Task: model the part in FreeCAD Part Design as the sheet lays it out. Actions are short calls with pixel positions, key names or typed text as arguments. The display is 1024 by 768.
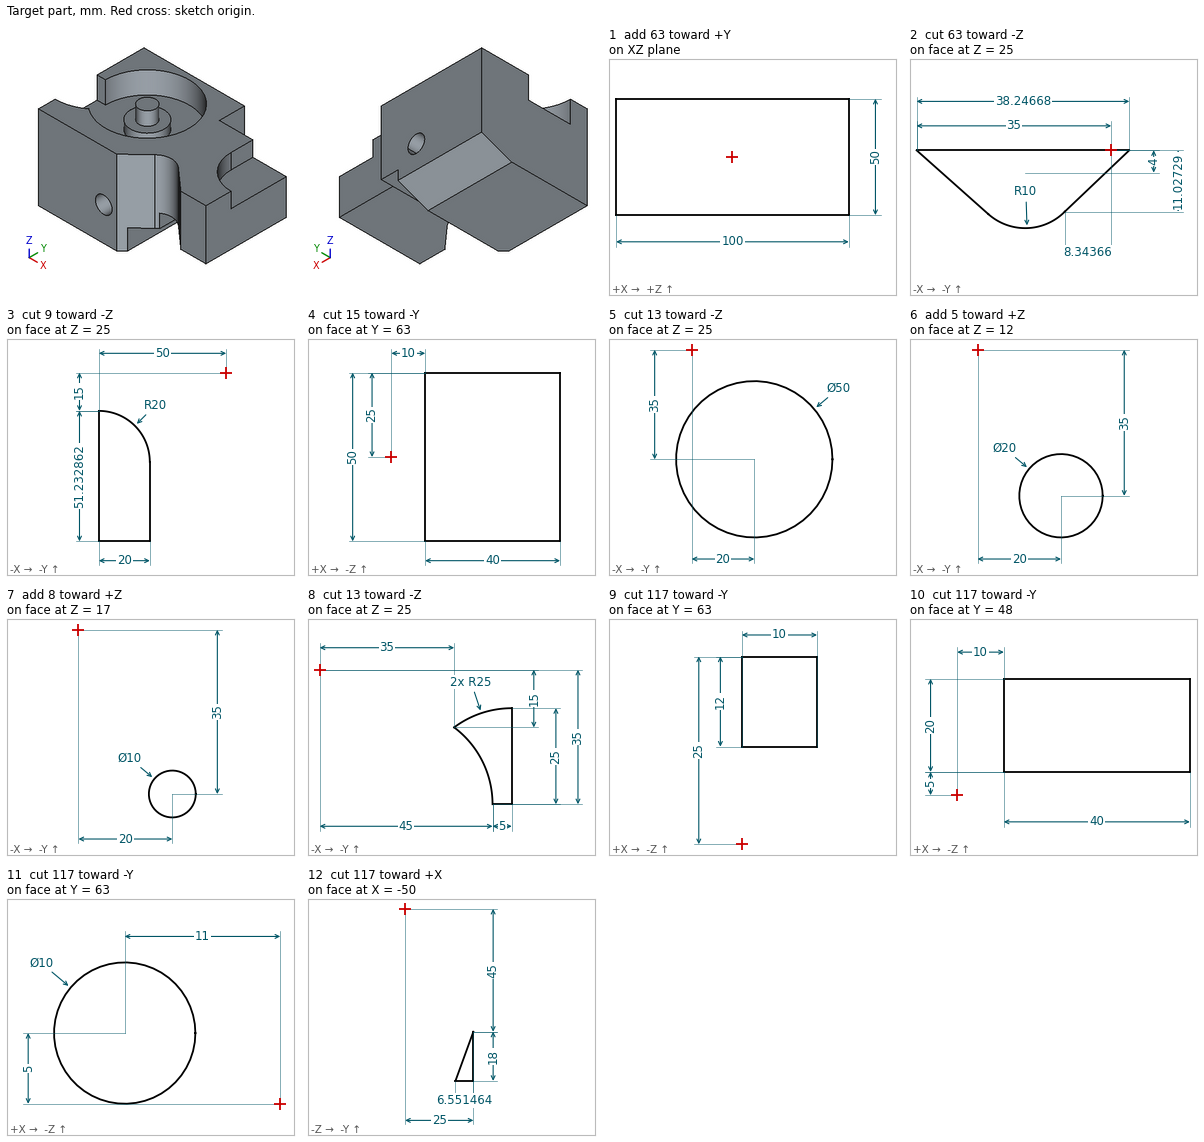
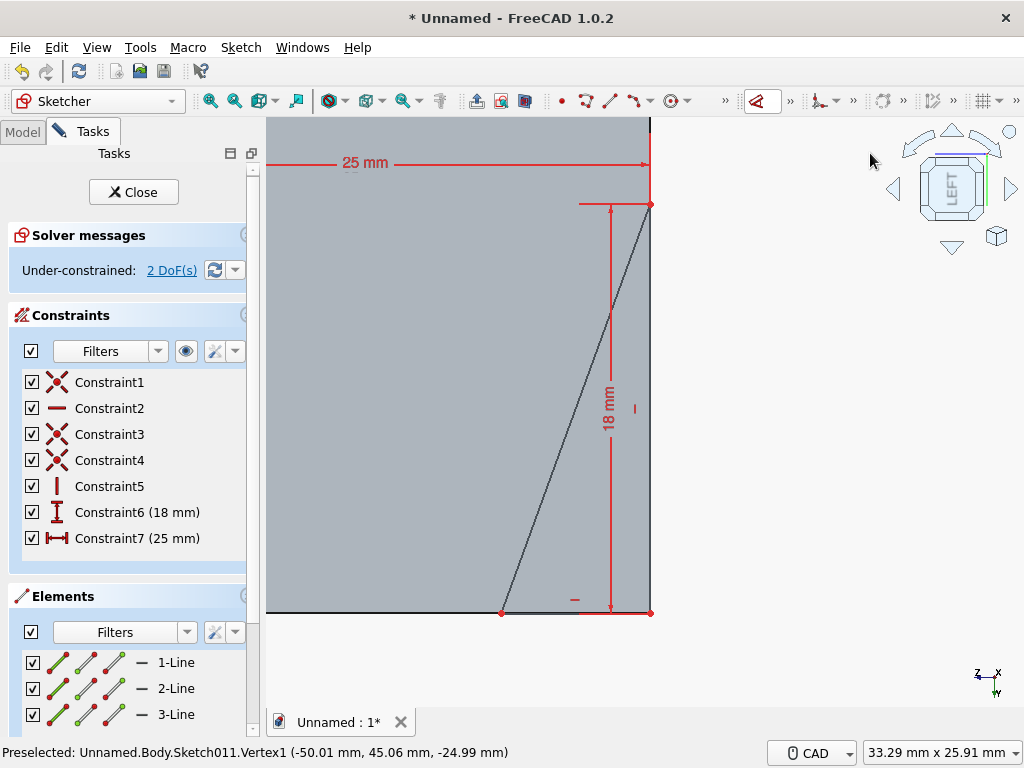
click(650, 204)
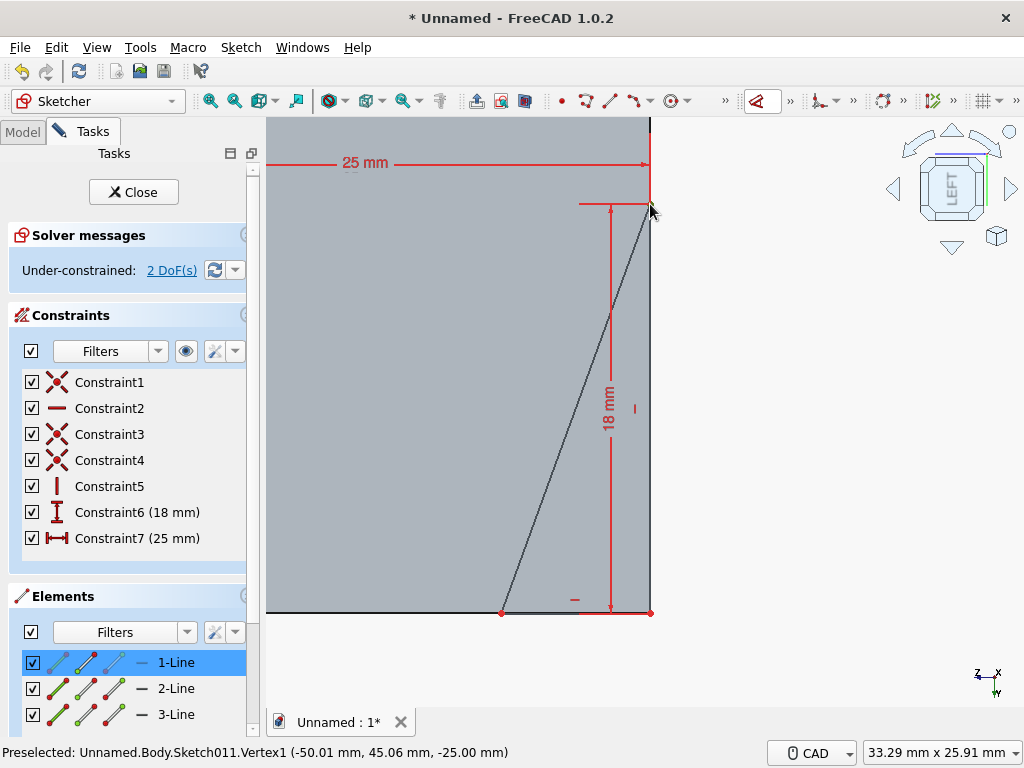
key(i)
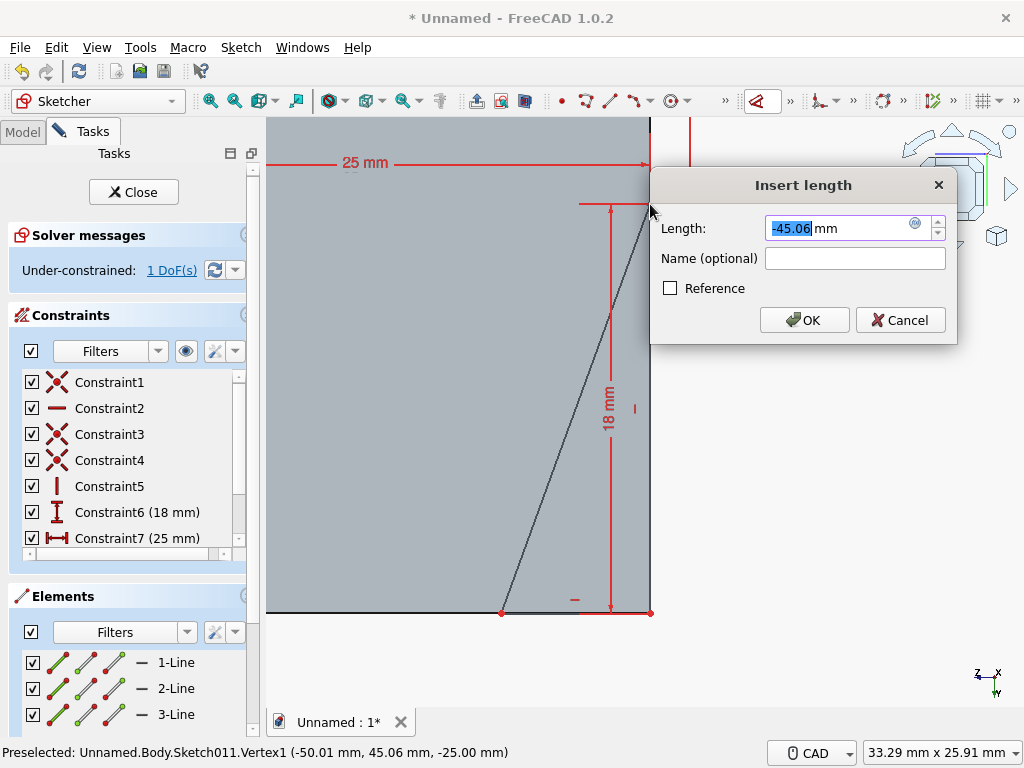
text(-45)
key(Return)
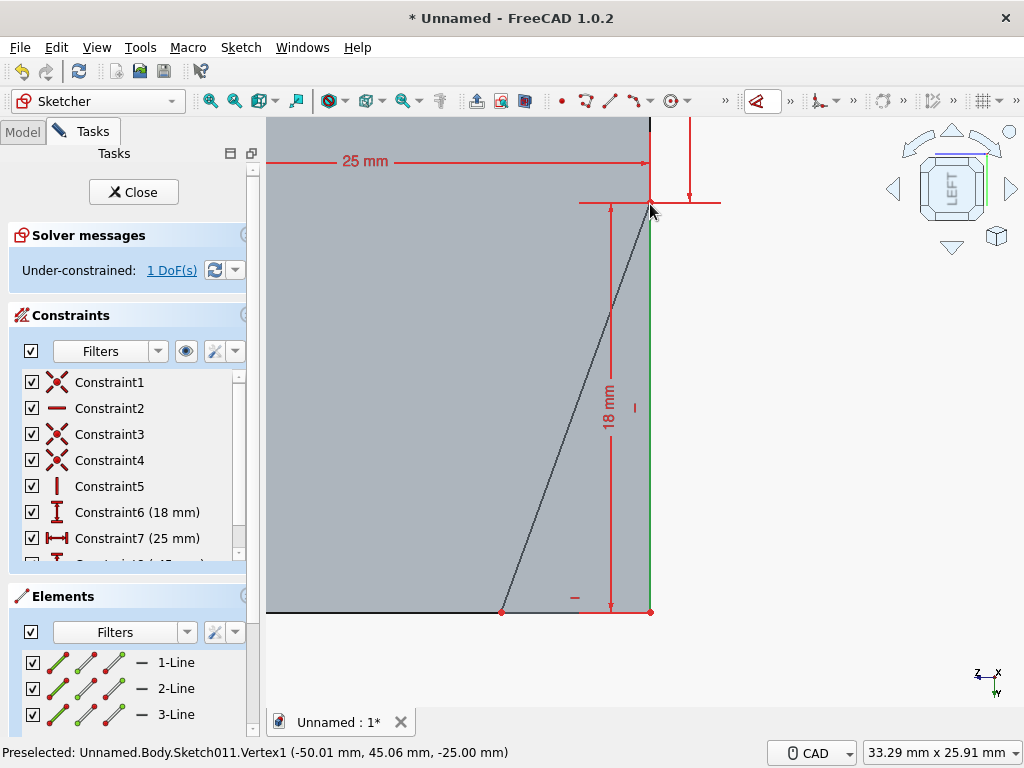
click(546, 613)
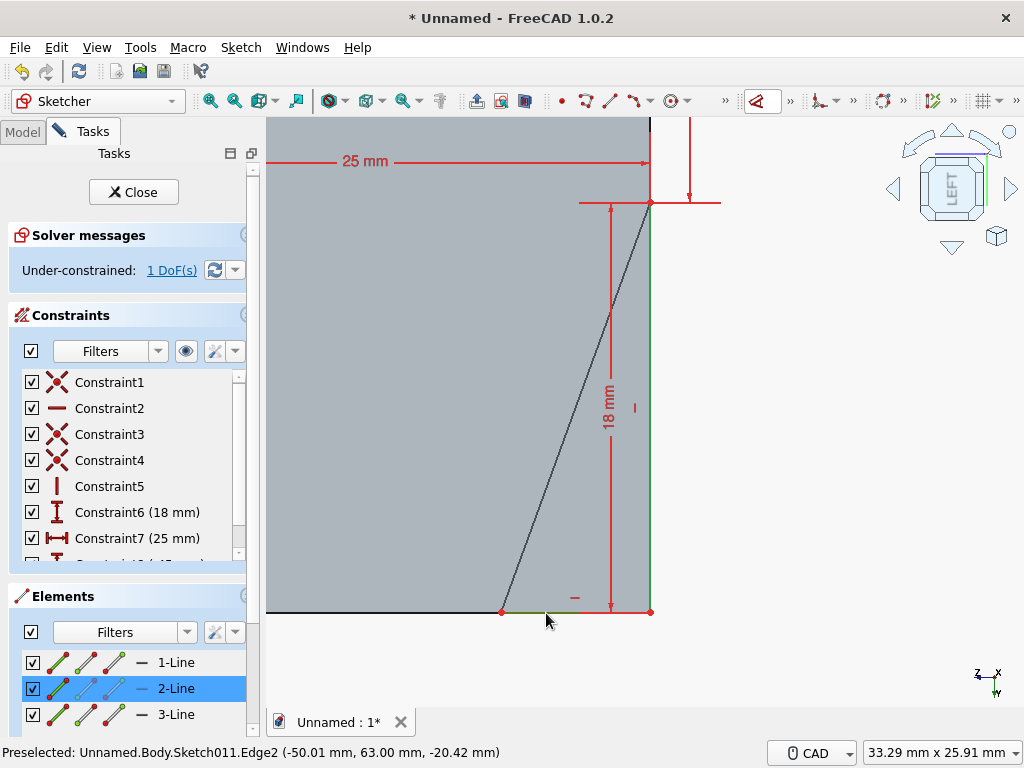
key(l)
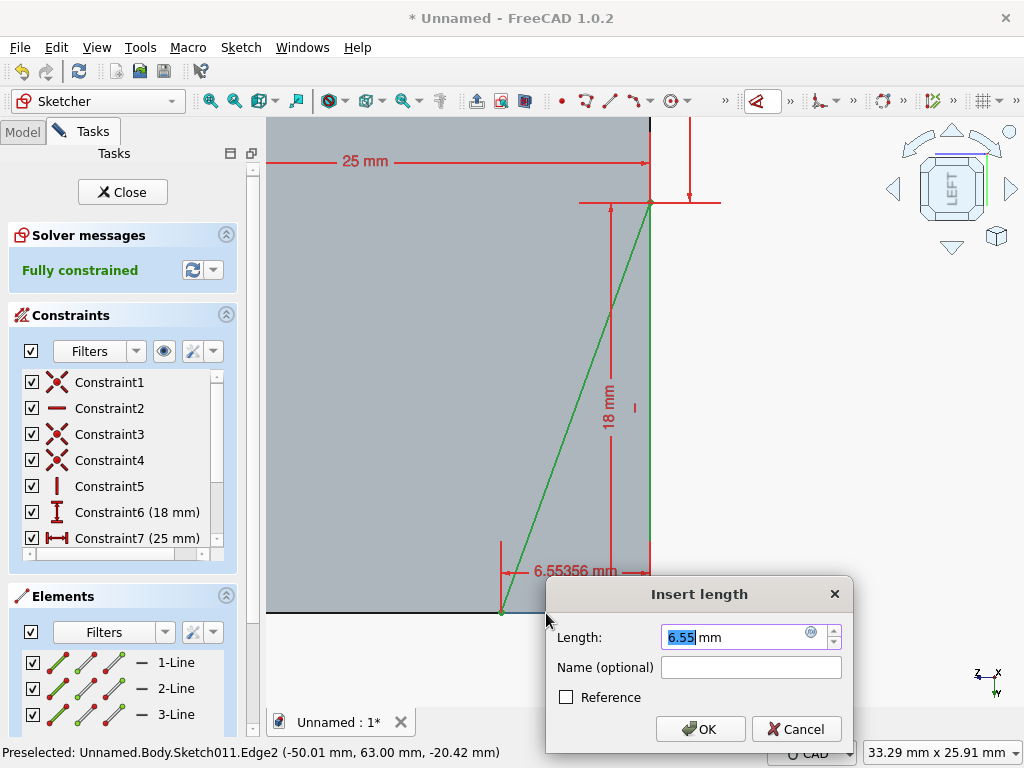
text(6.551464)
key(Return)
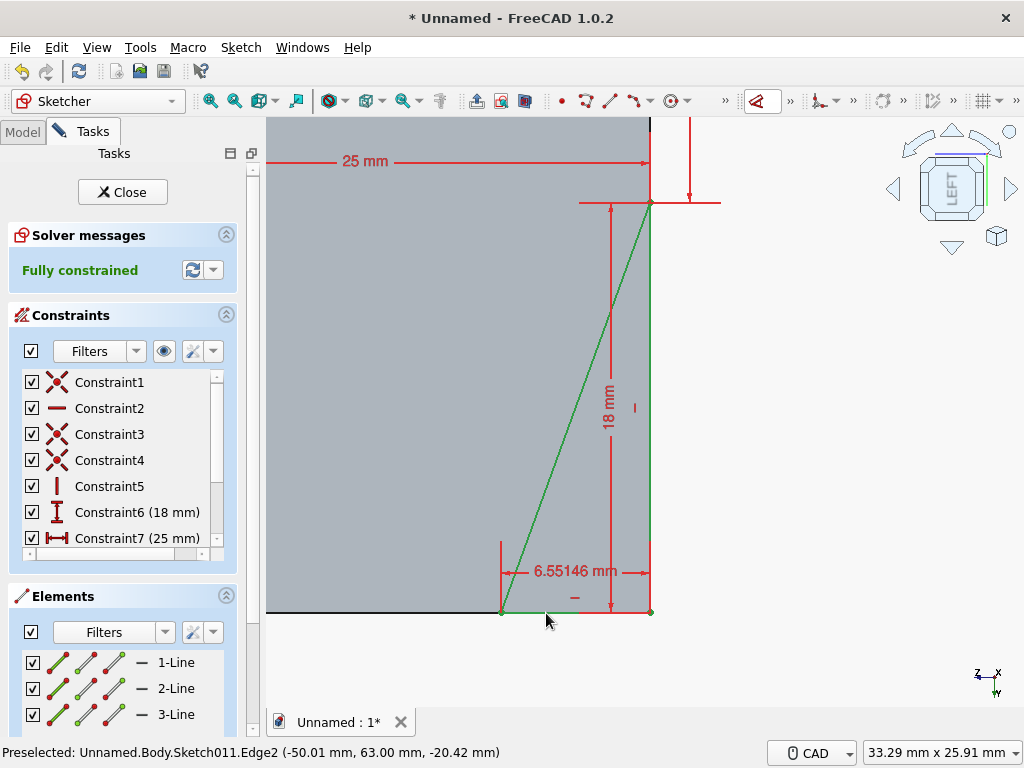
click(123, 192)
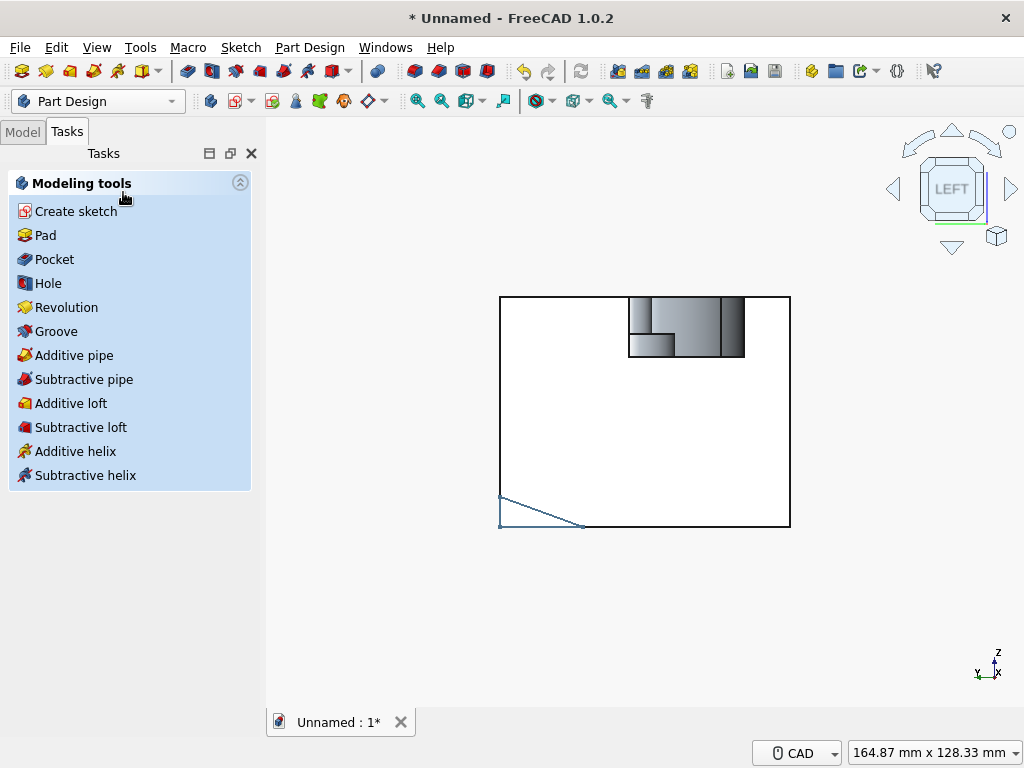
click(188, 72)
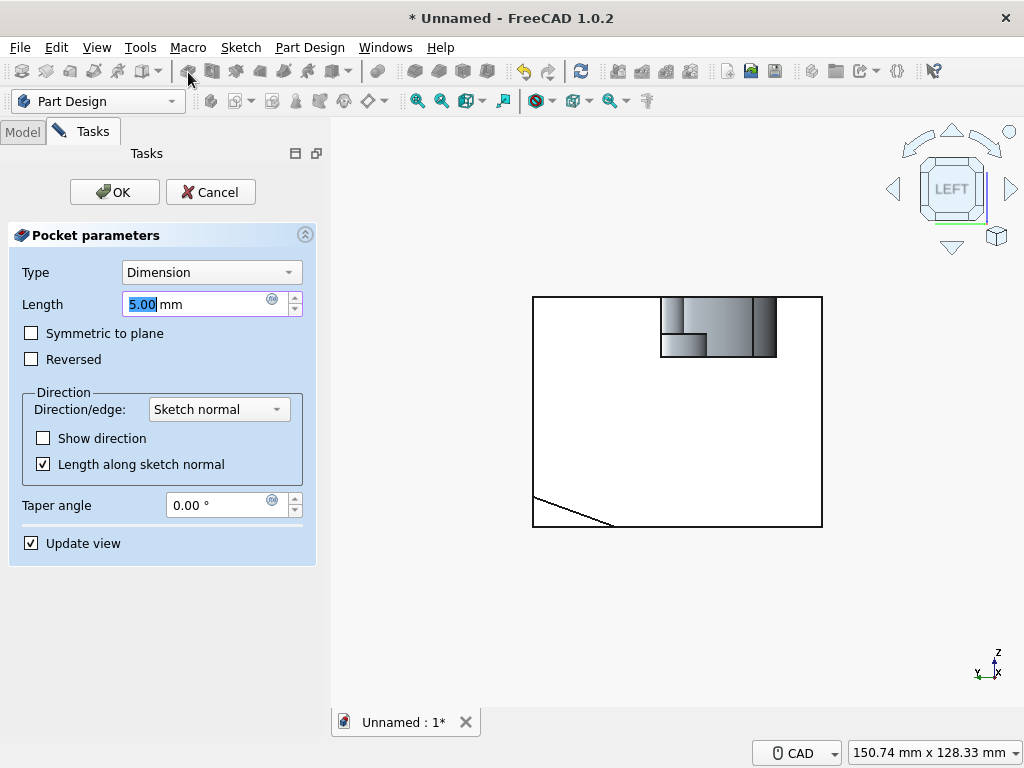
text(117)
key(Tab)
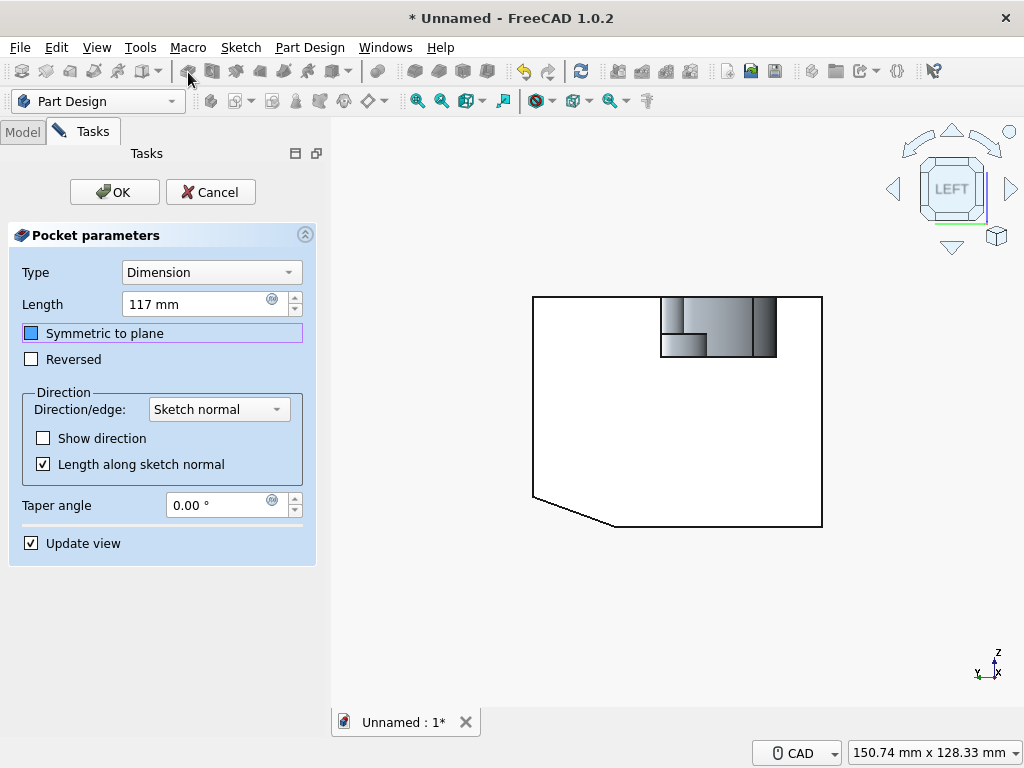
click(115, 192)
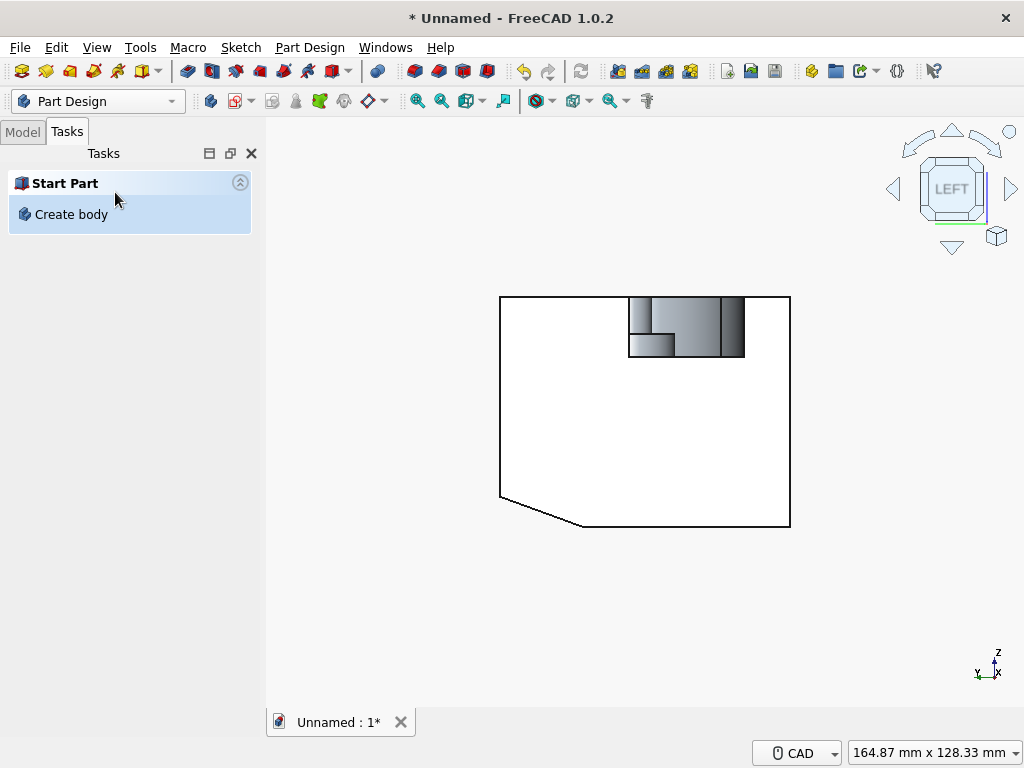
key(0)